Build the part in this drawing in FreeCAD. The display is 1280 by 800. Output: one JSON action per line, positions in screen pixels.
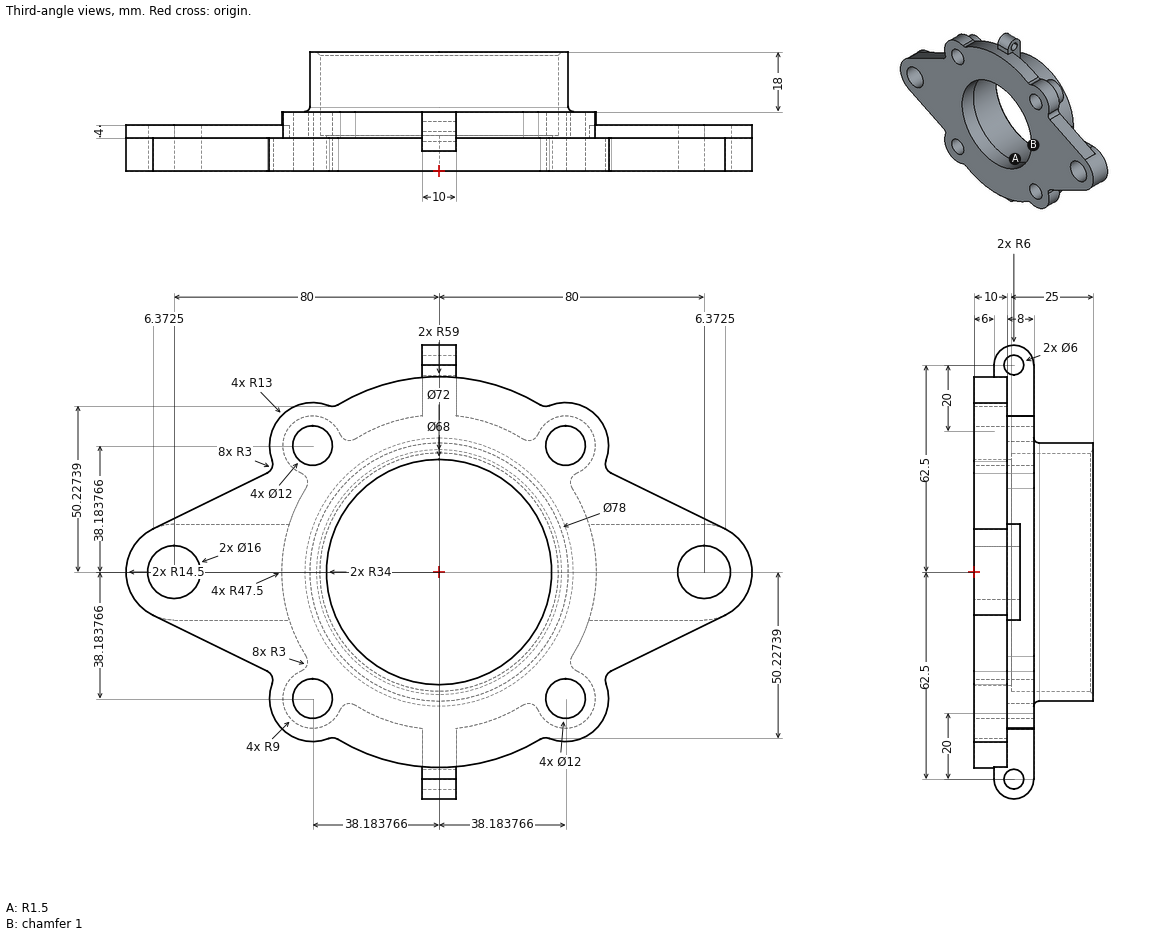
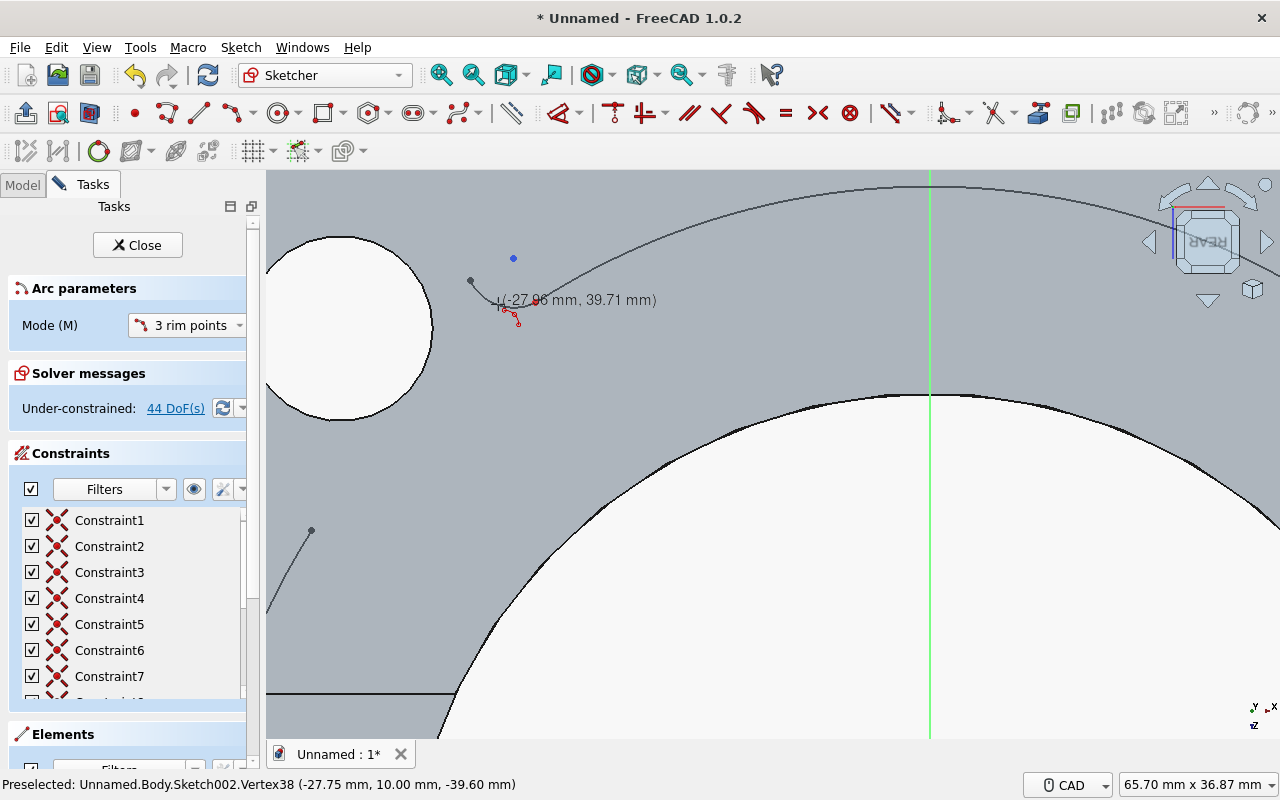
{"action": "scroll", "coordinate": [631, 303], "scroll_direction": "down", "scroll_amount": 7}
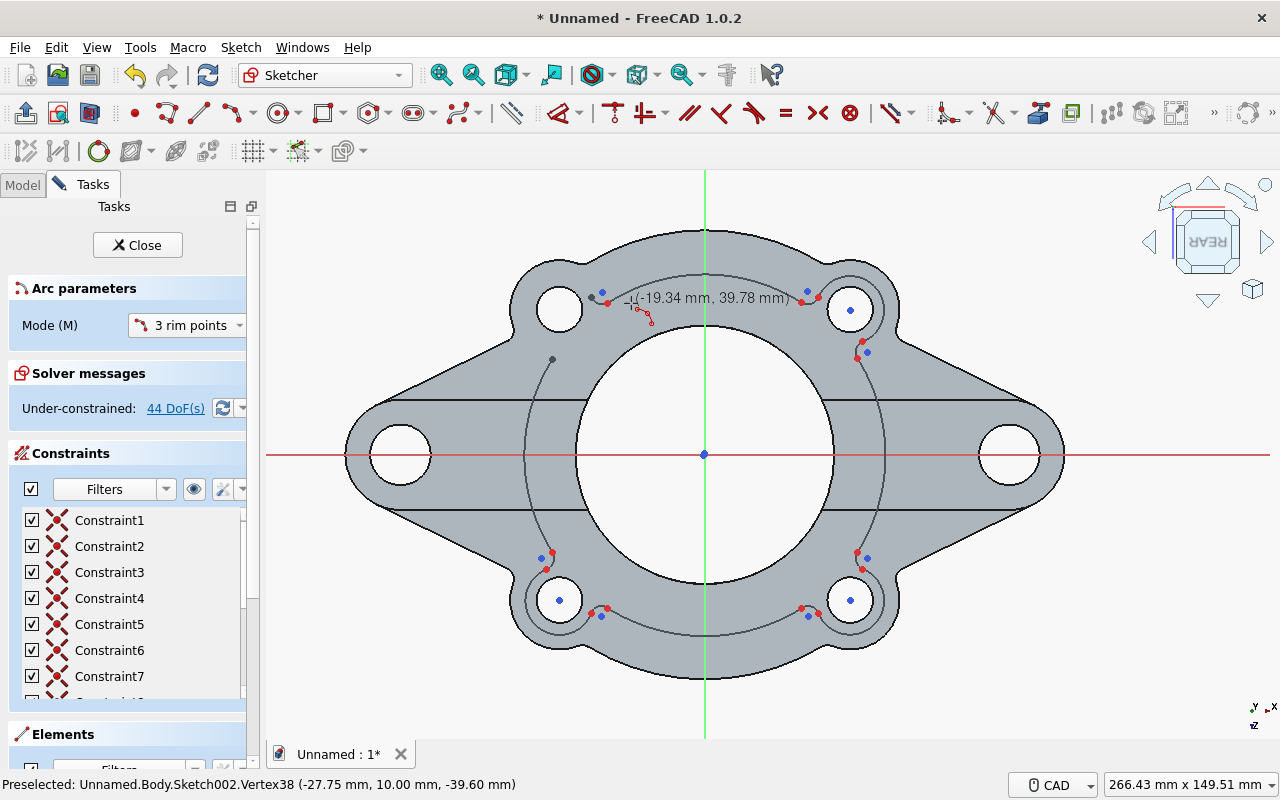
{"action": "scroll", "coordinate": [591, 297], "scroll_direction": "up", "scroll_amount": 2}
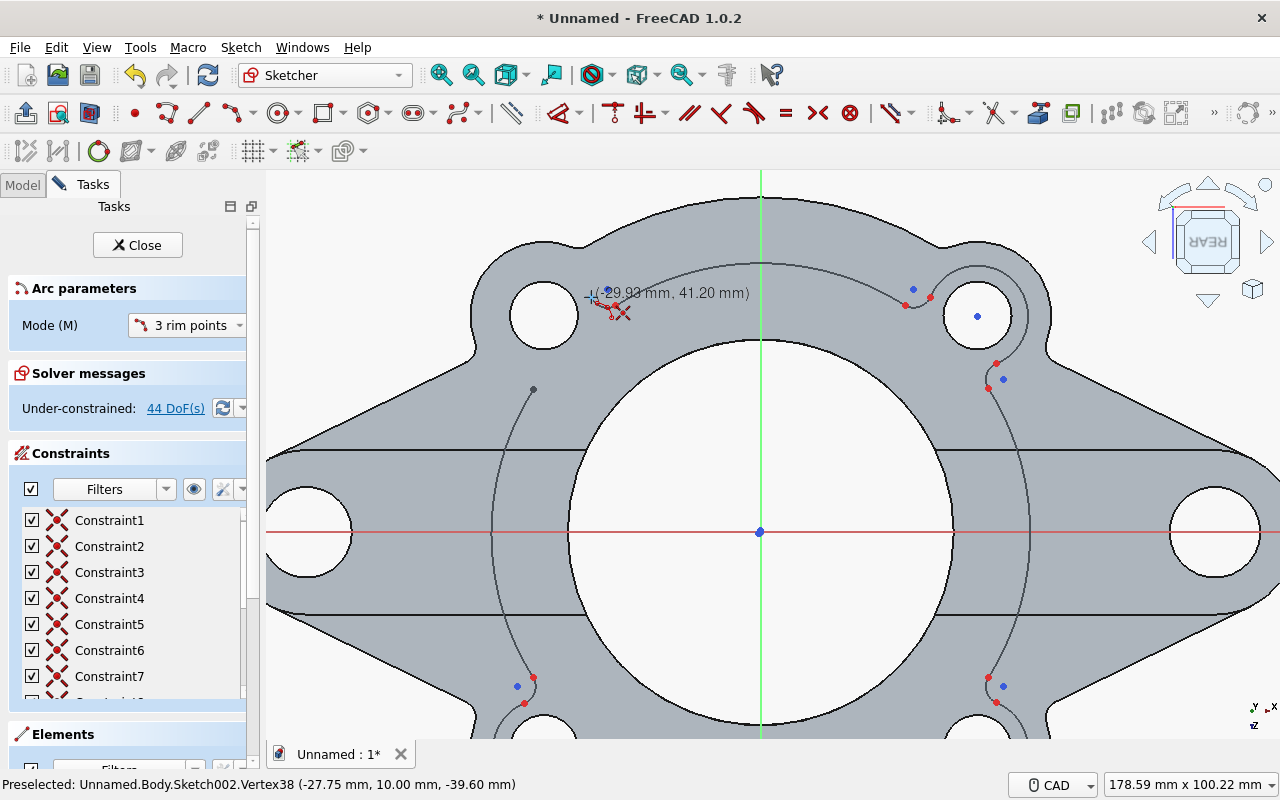
{"action": "left_click", "coordinate": [592, 298]}
{"action": "left_click", "coordinate": [525, 363]}
{"action": "left_click", "coordinate": [508, 279]}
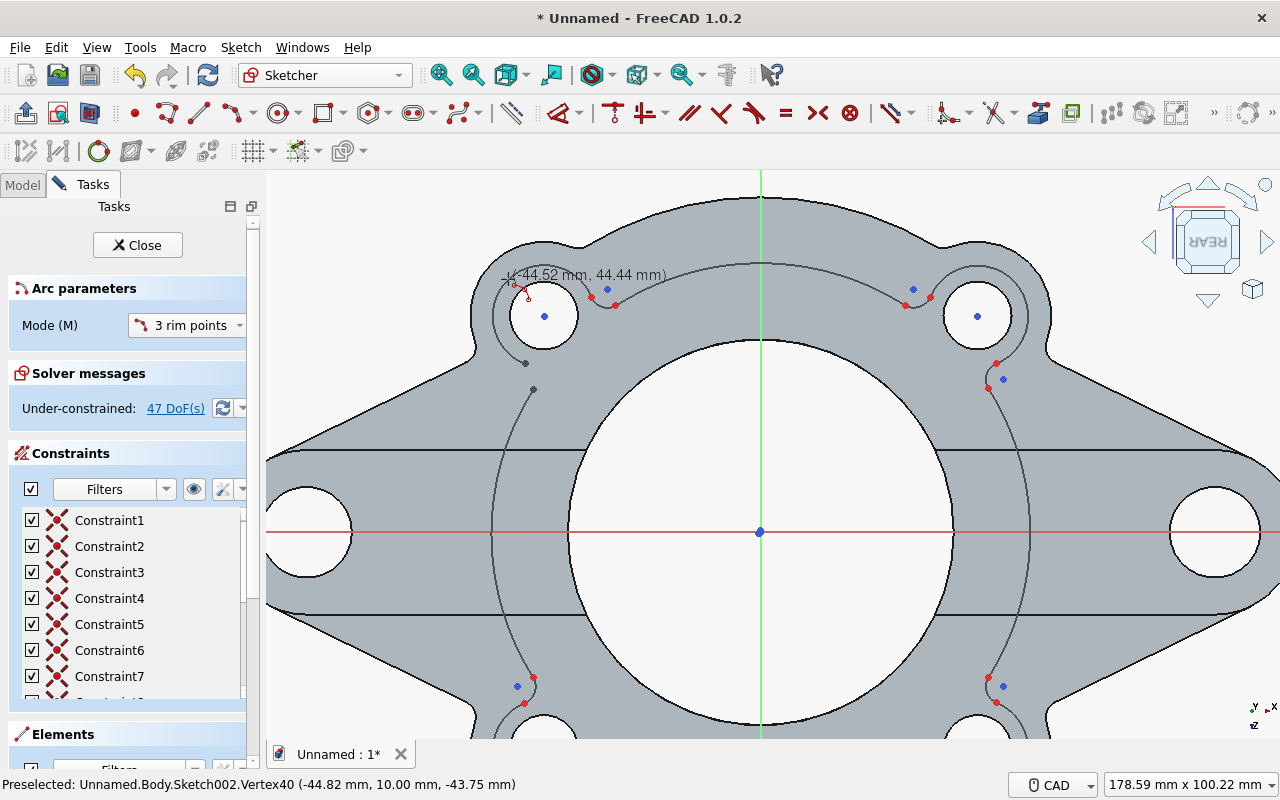
{"action": "left_click", "coordinate": [525, 364]}
{"action": "left_click", "coordinate": [534, 390]}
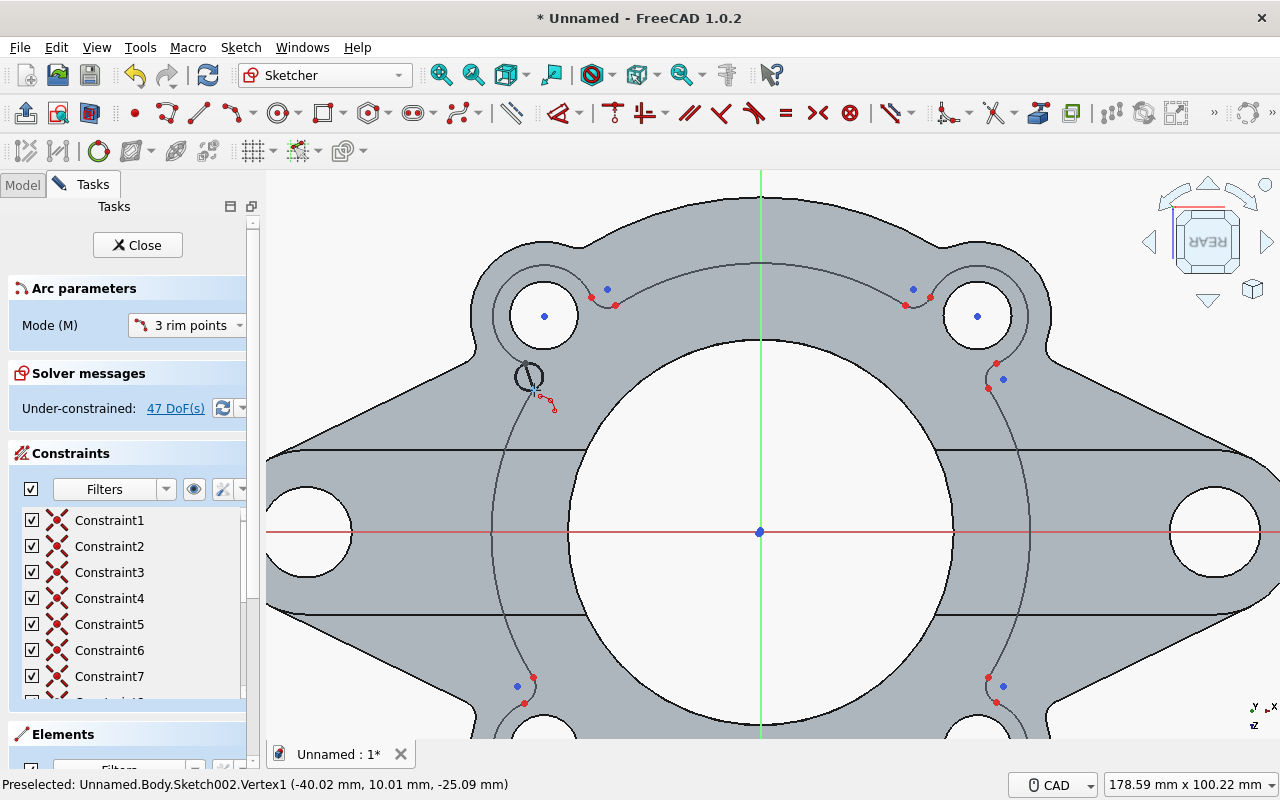
{"action": "scroll", "coordinate": [535, 374], "scroll_direction": "up", "scroll_amount": 5}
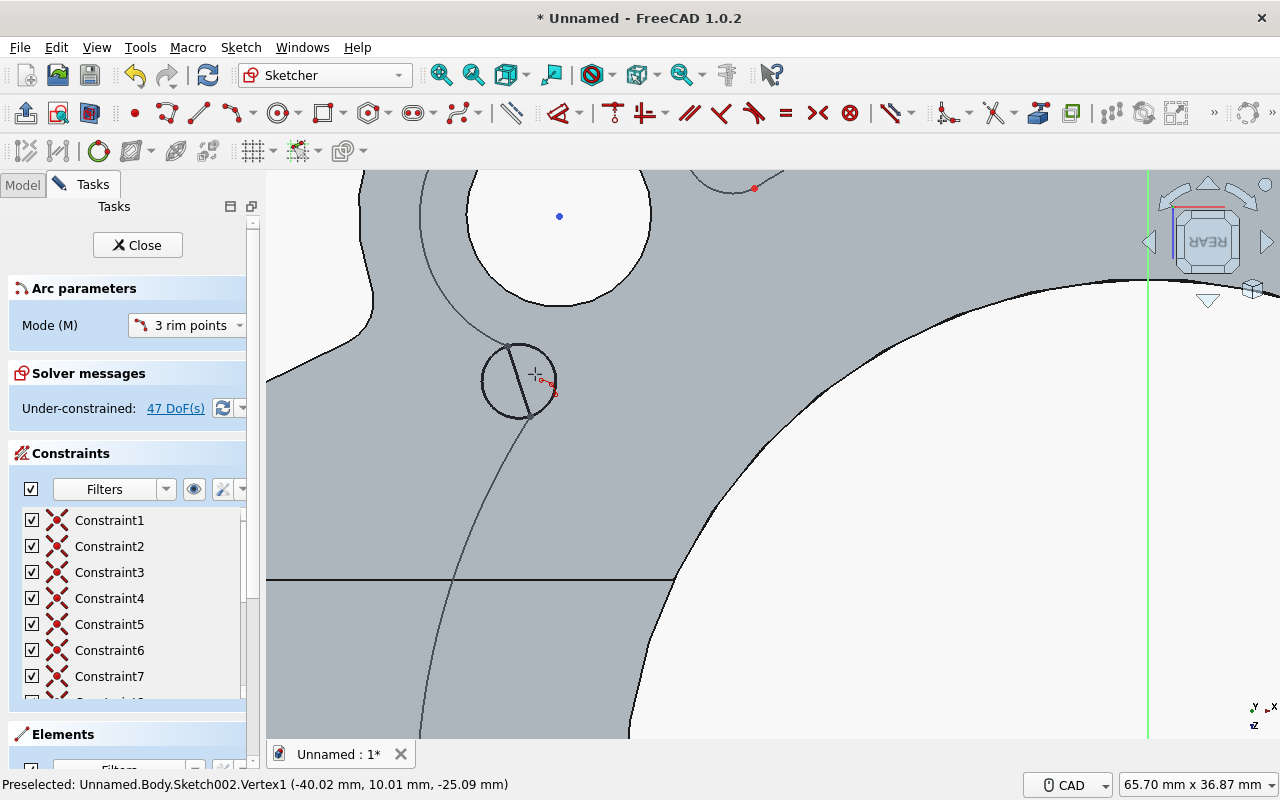
{"action": "left_click", "coordinate": [534, 372]}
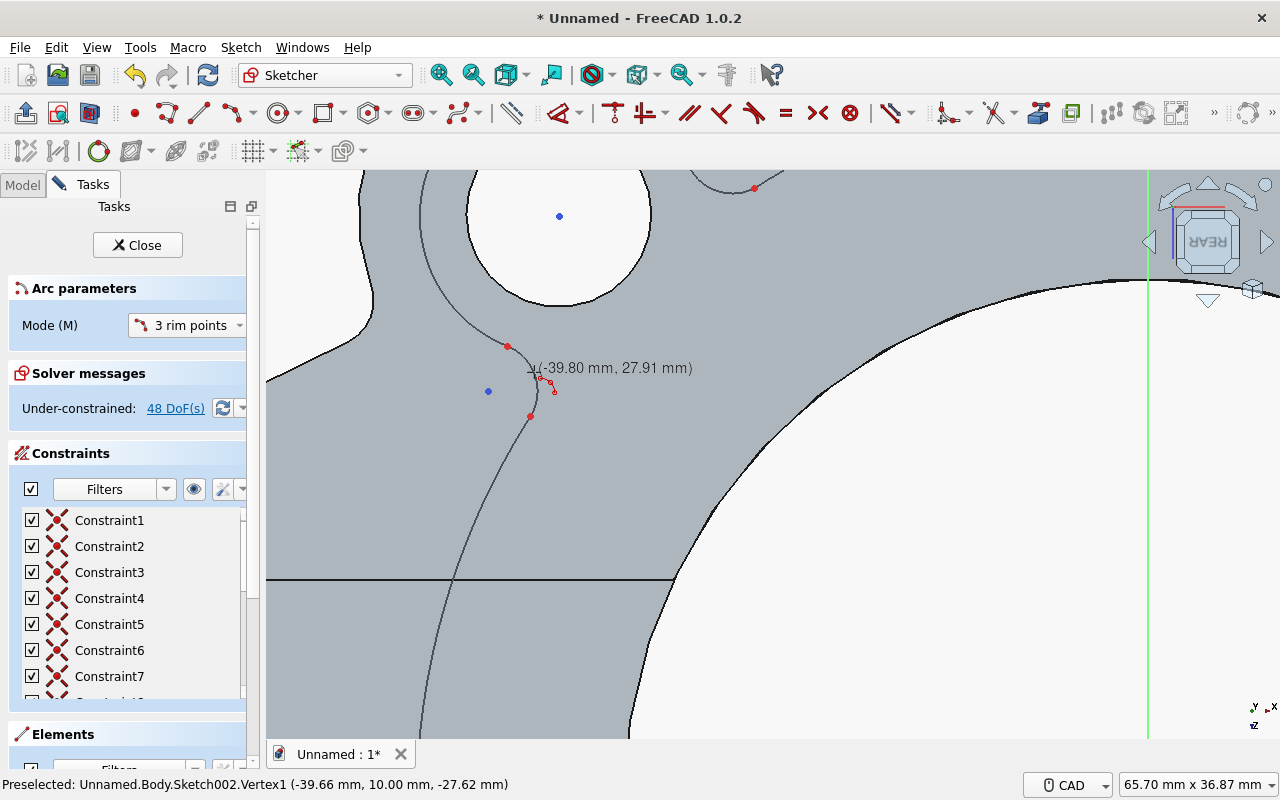
{"action": "left_click", "coordinate": [278, 114]}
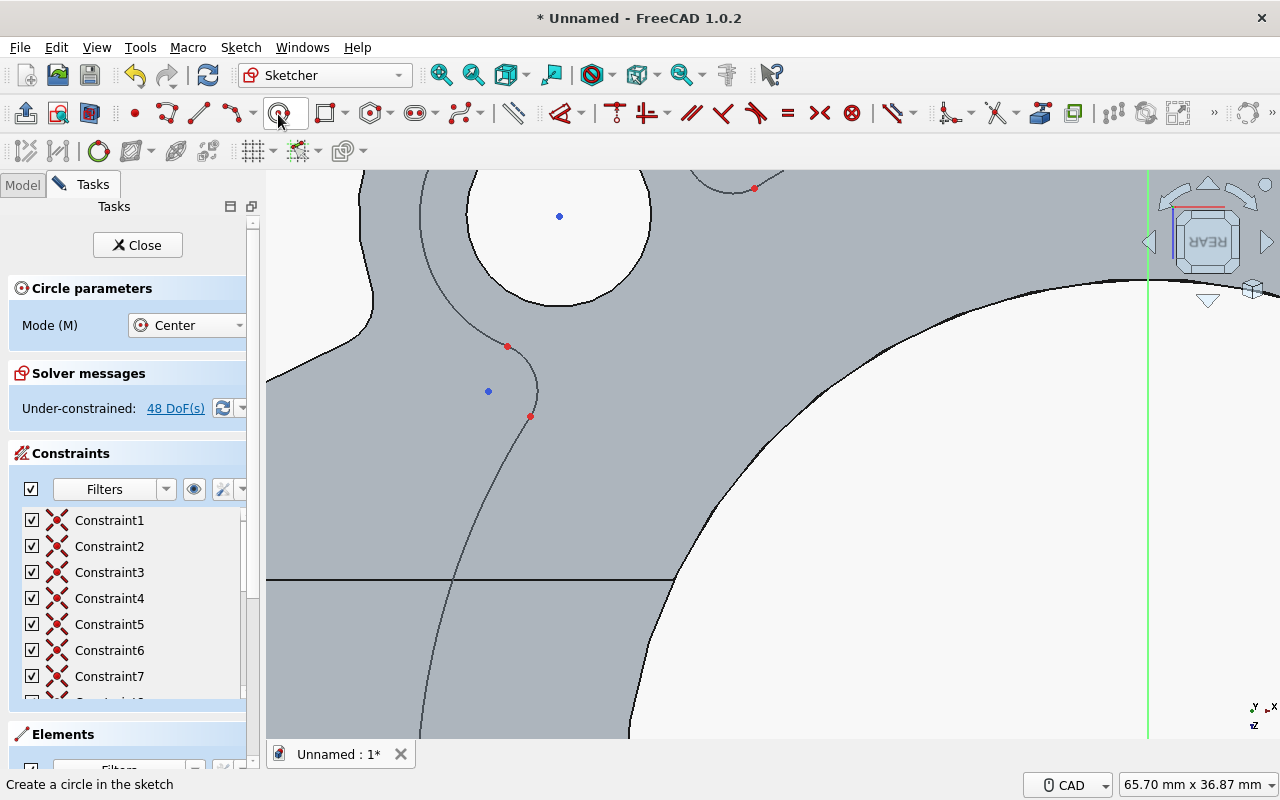
{"action": "scroll", "coordinate": [559, 340], "scroll_direction": "down", "scroll_amount": 7}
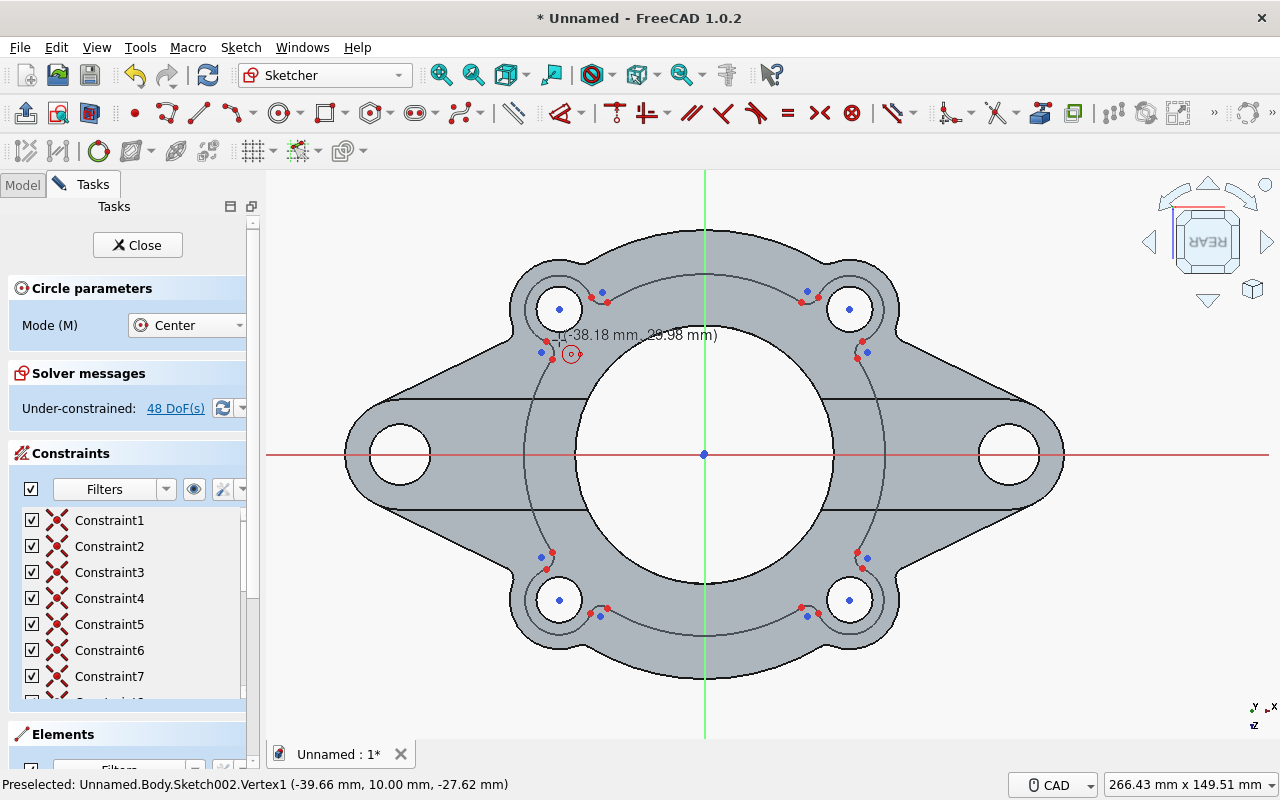
{"action": "left_click", "coordinate": [559, 600]}
{"action": "mouse_move", "coordinate": [575, 584]}